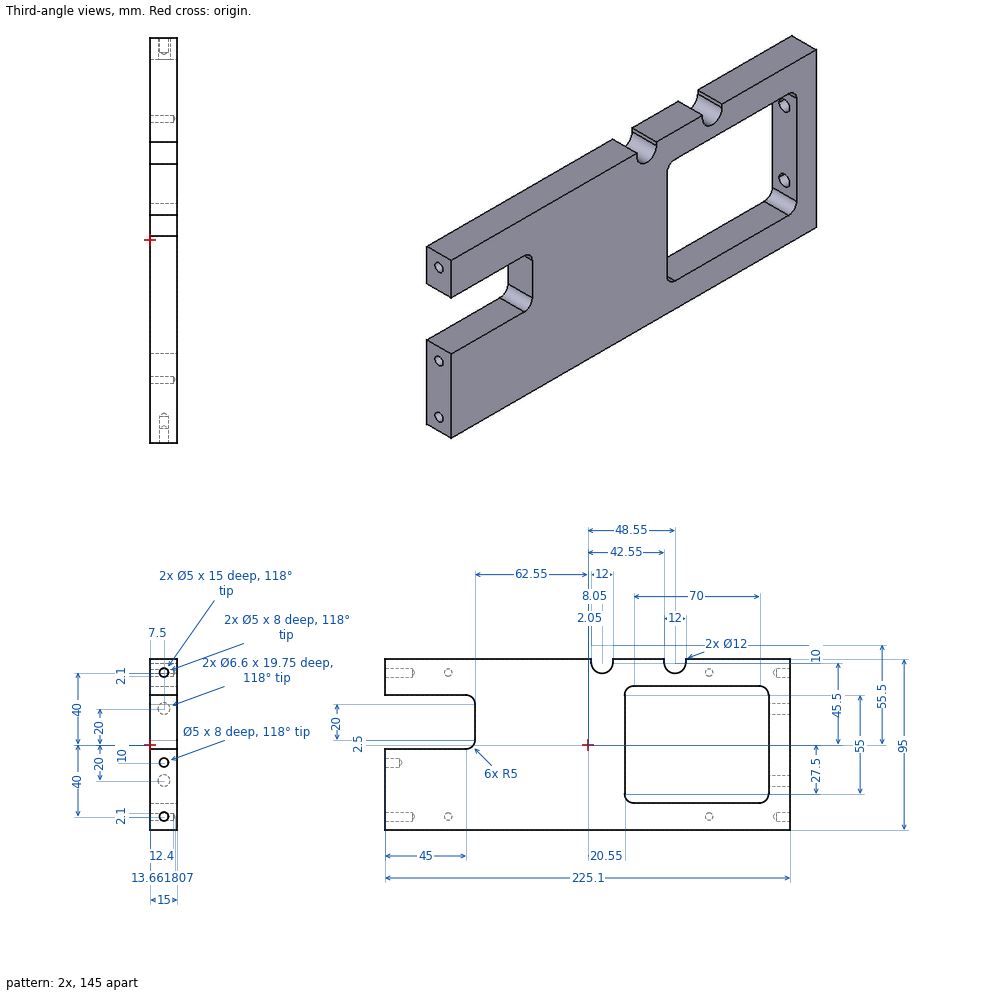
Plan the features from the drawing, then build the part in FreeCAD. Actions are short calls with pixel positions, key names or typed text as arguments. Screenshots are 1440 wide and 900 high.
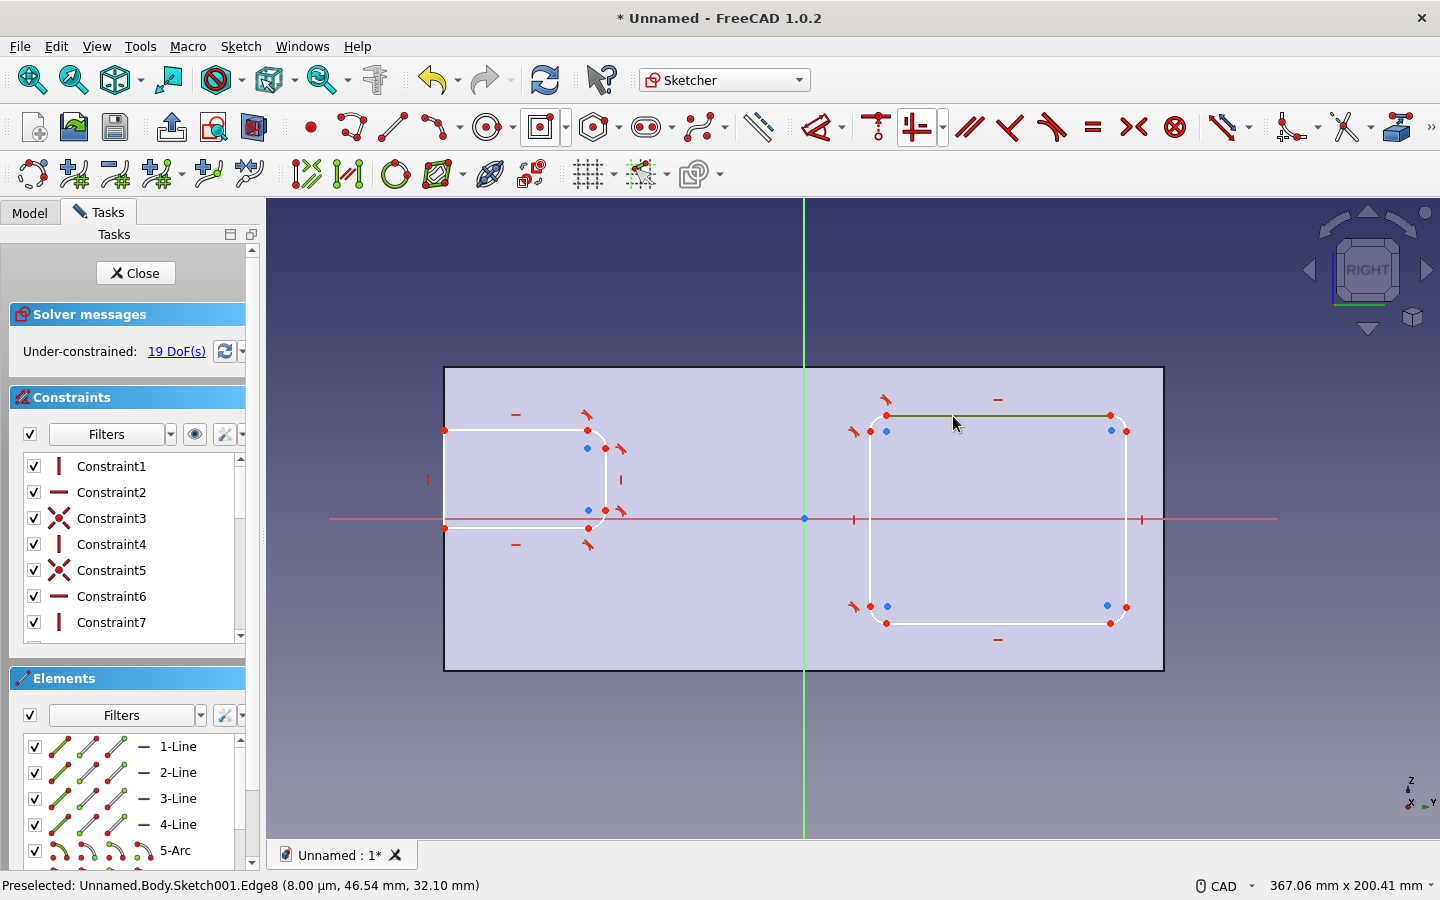
click(1122, 420)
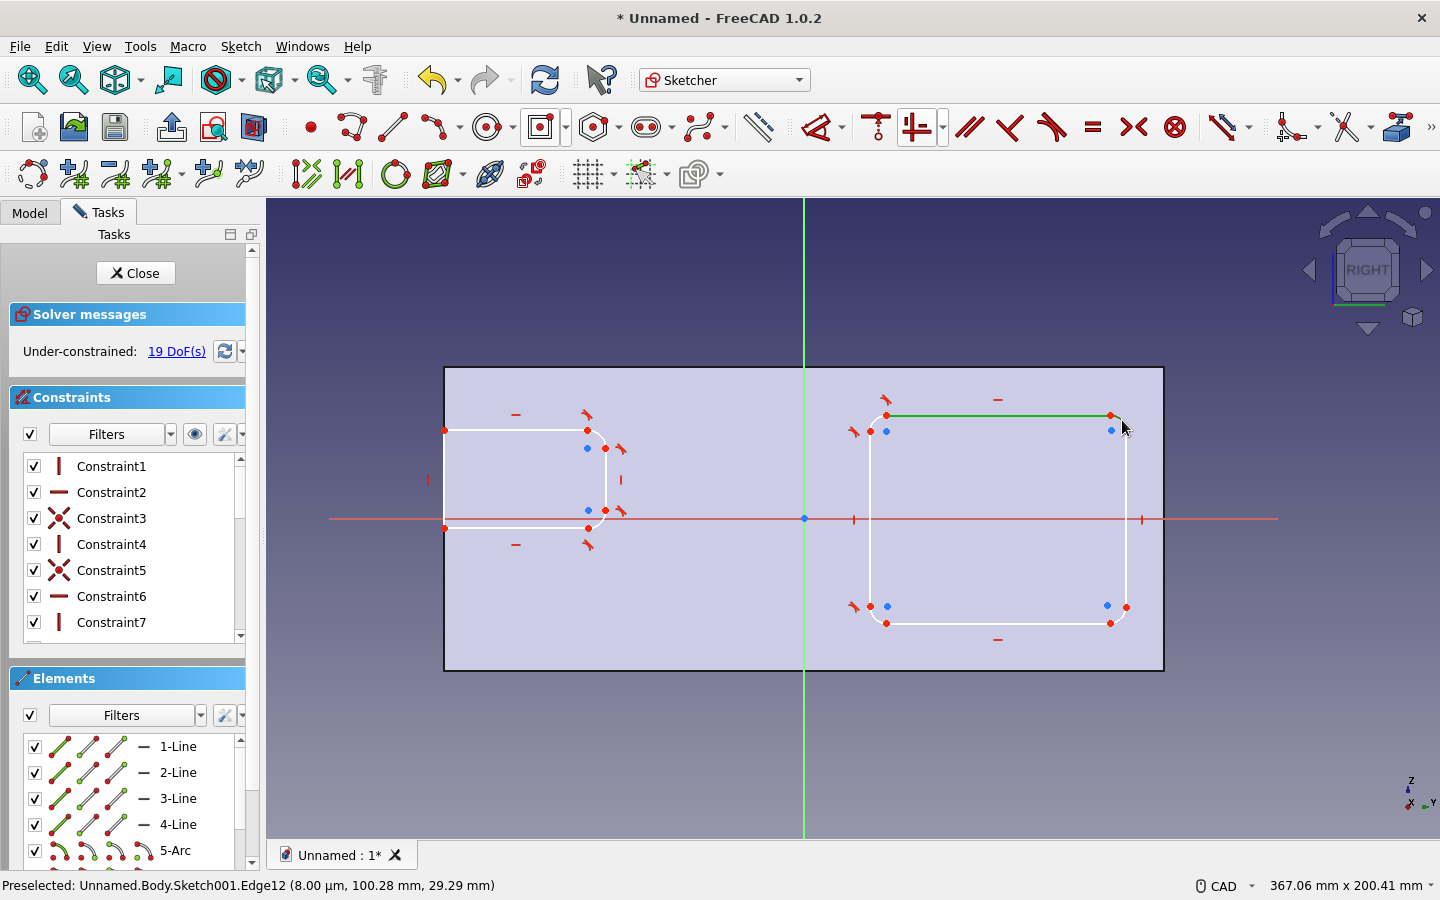
click(1052, 128)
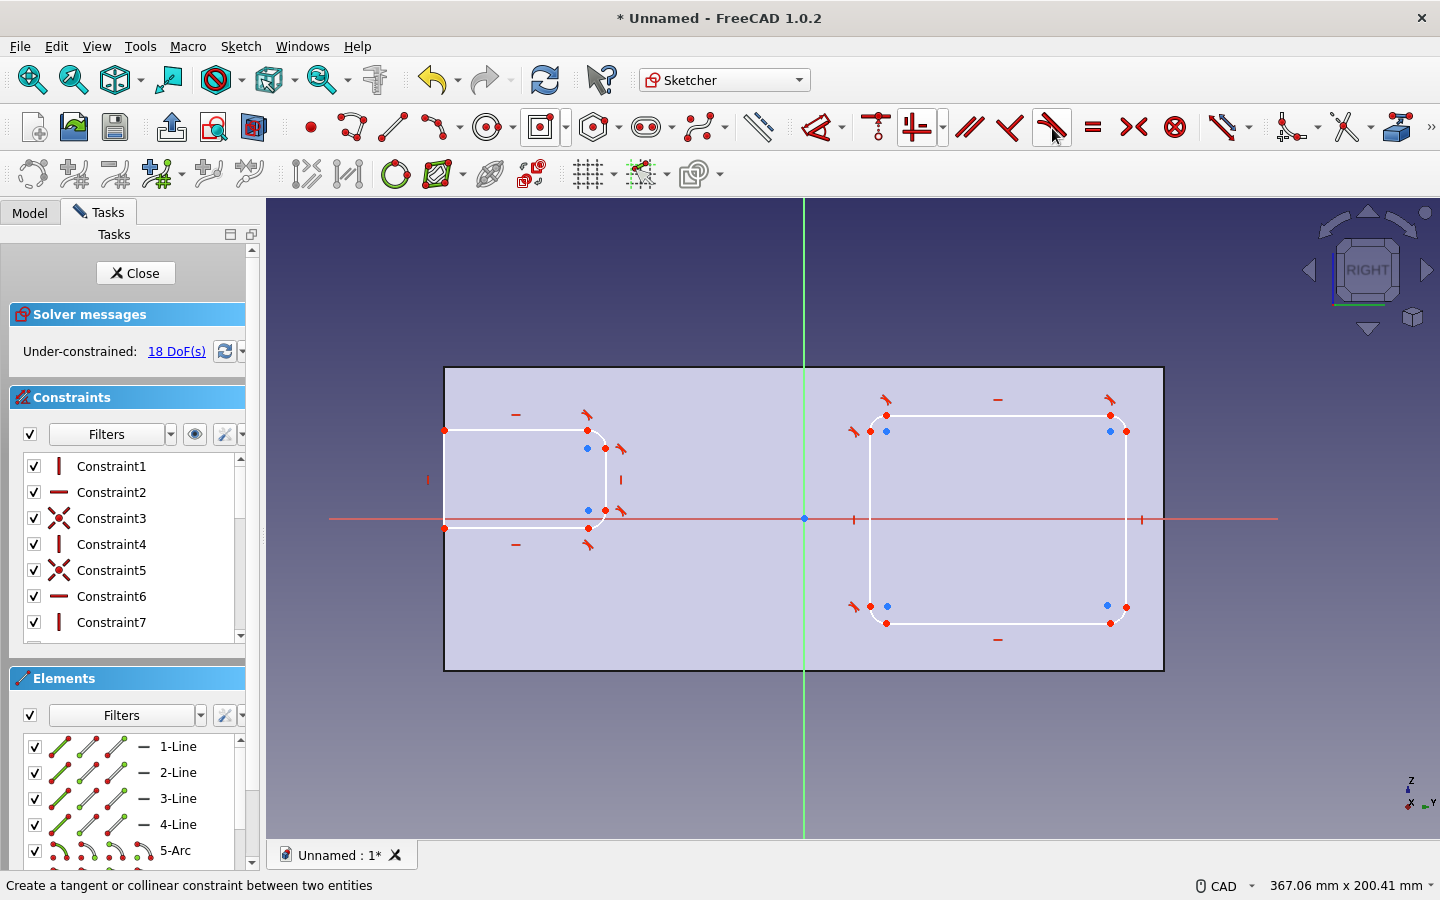
click(1126, 485)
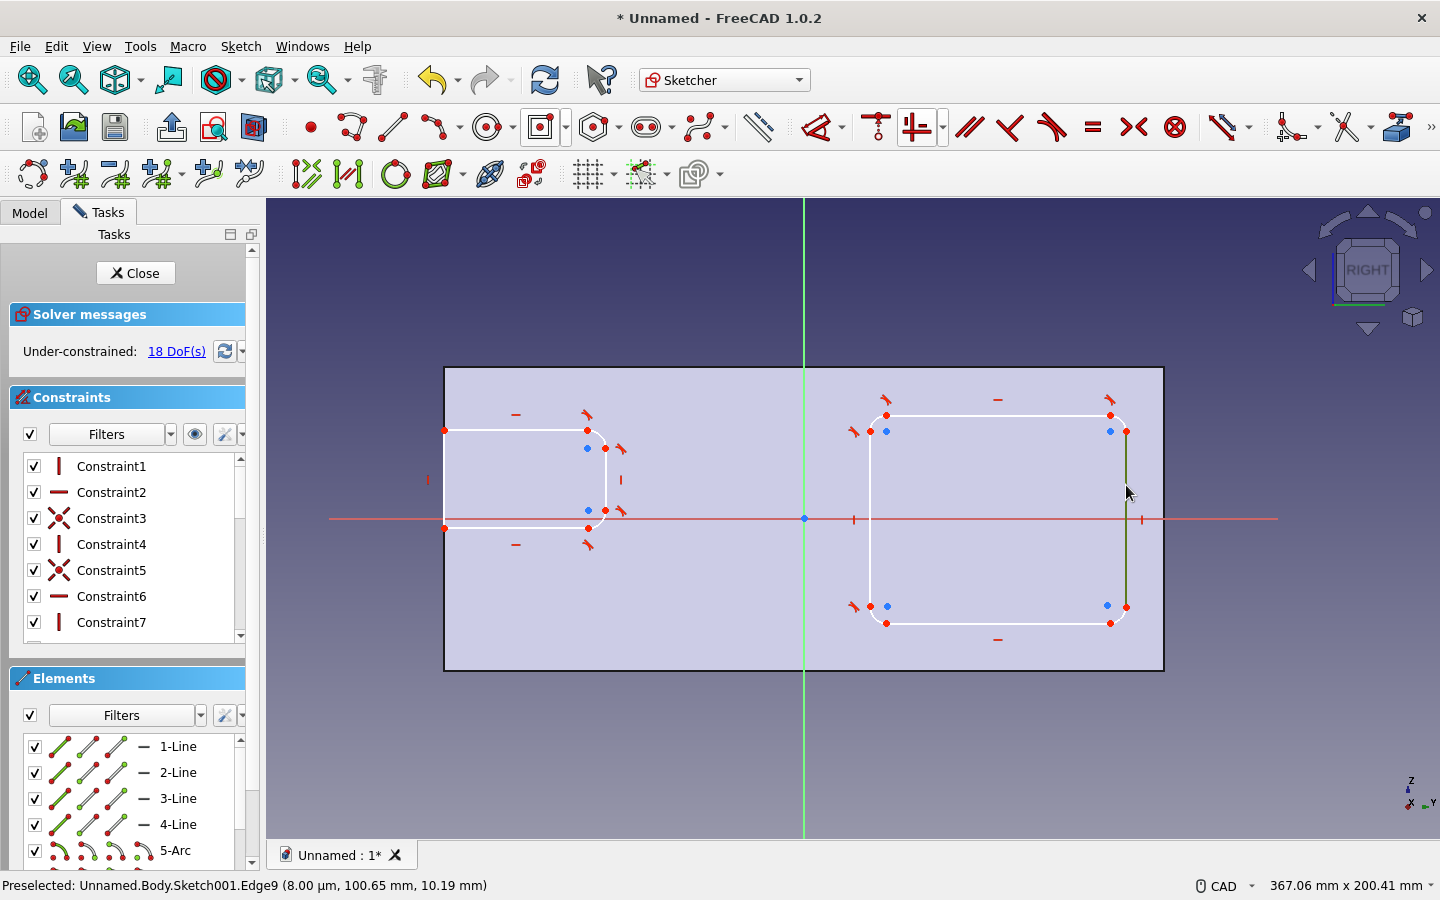
click(1121, 421)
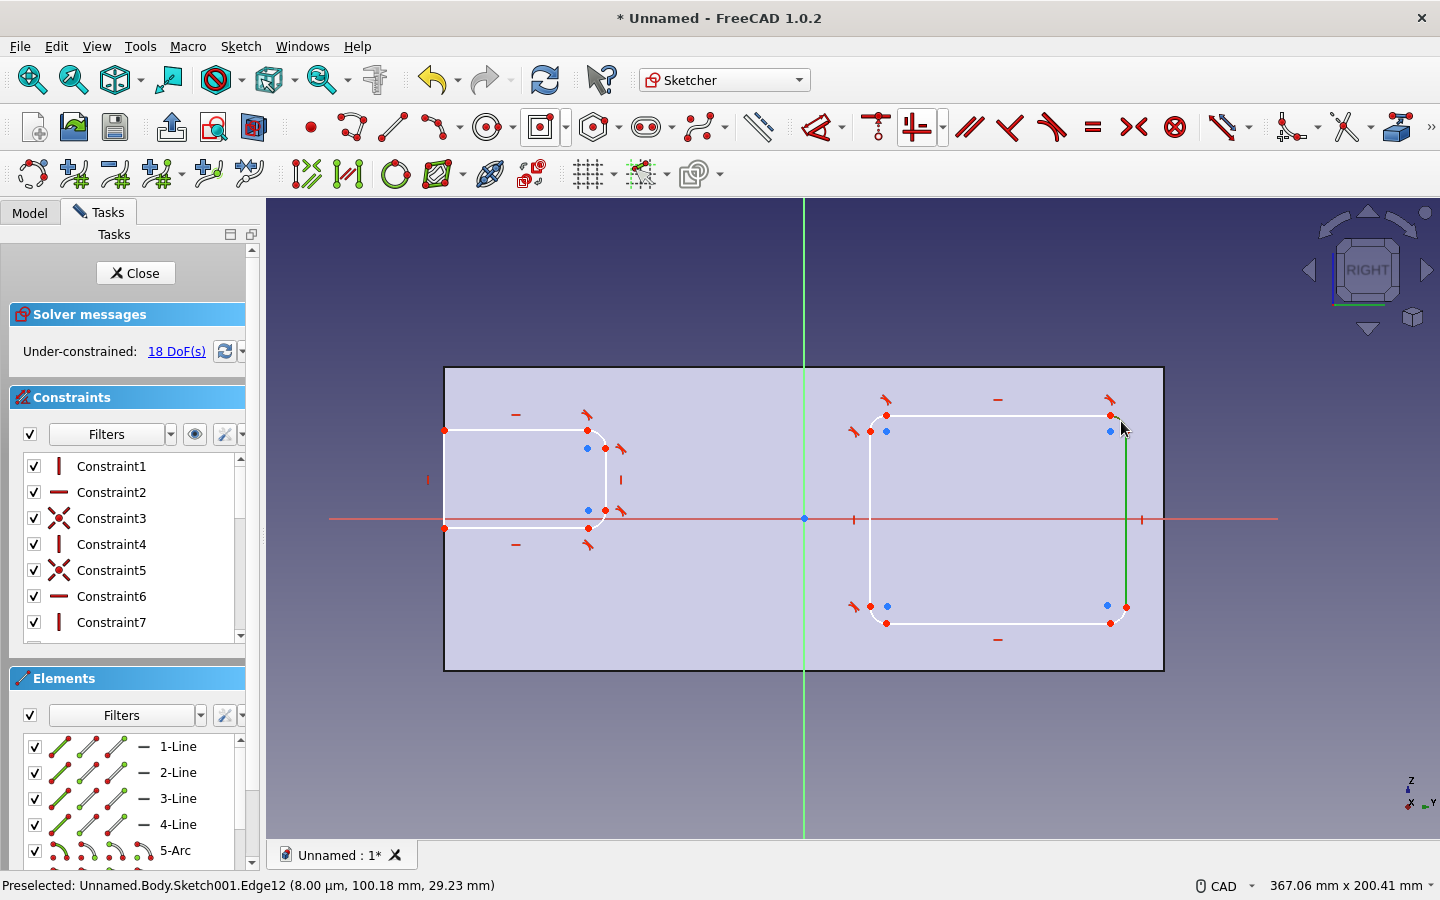
click(1052, 128)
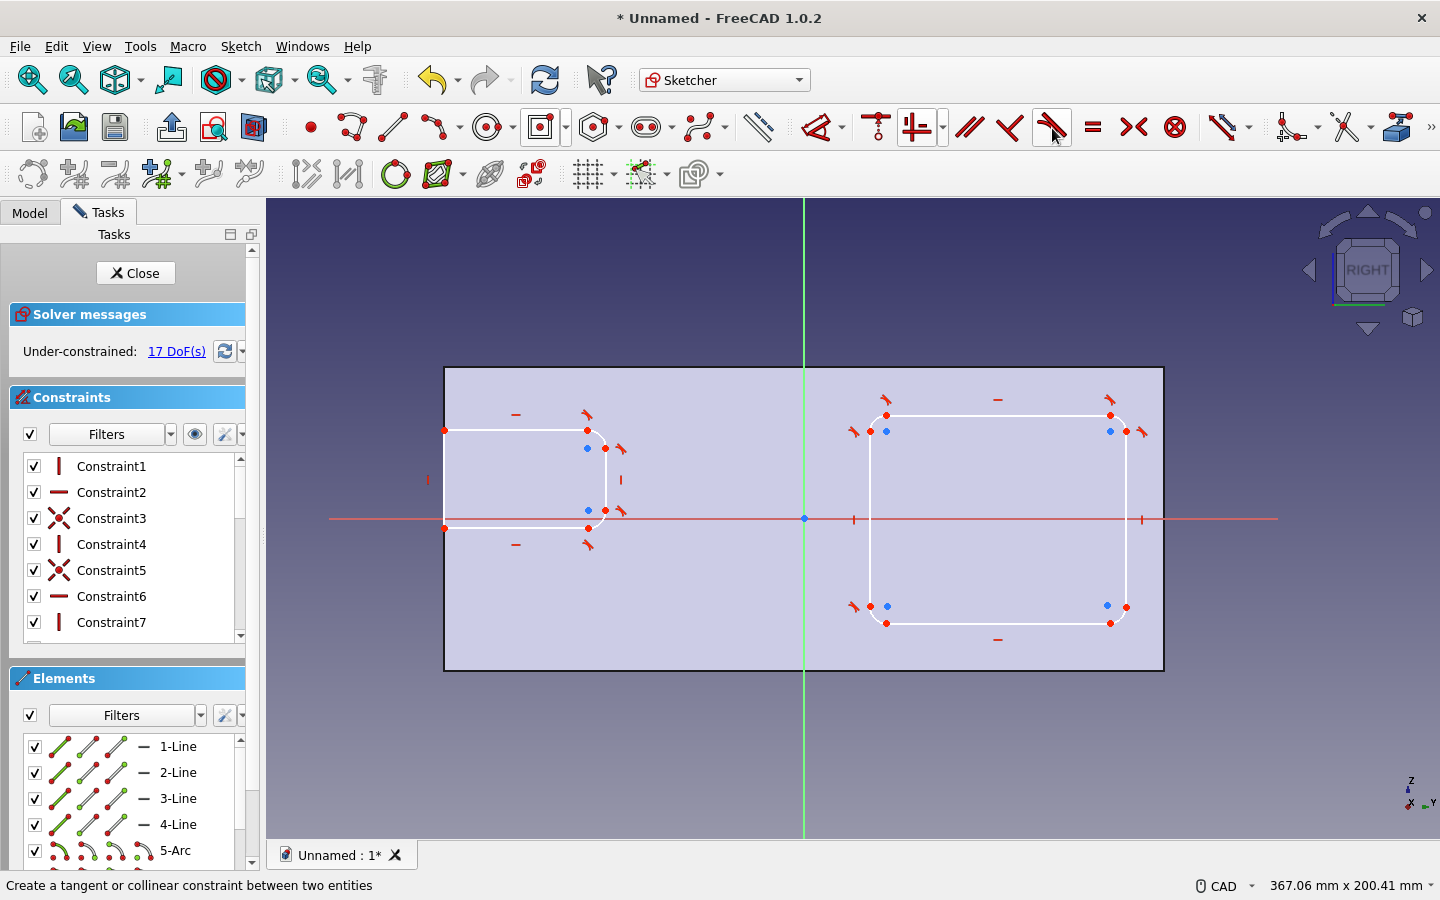
click(1126, 485)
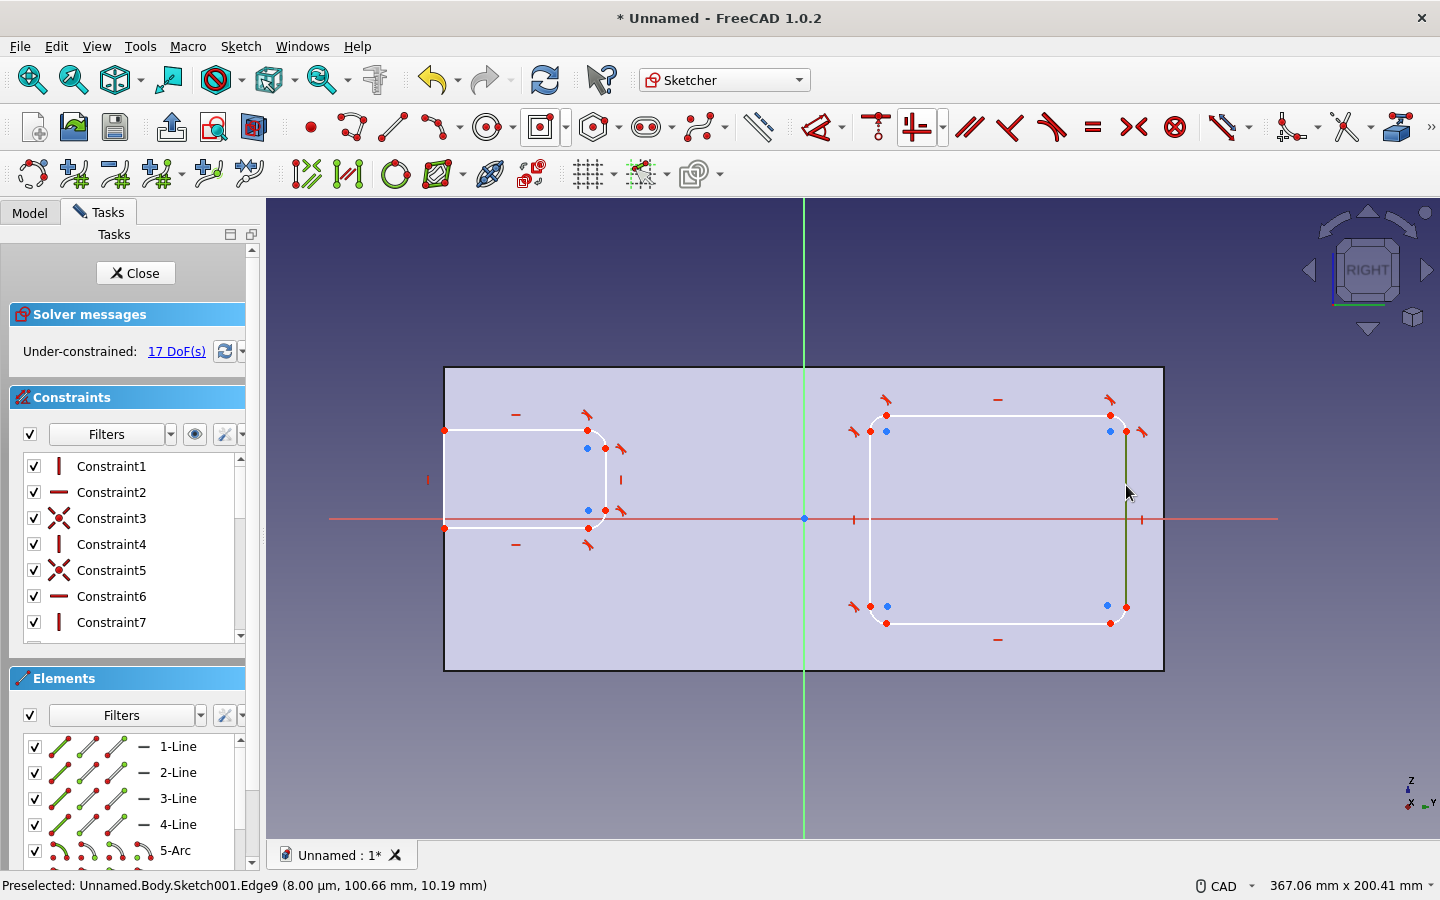
click(1121, 619)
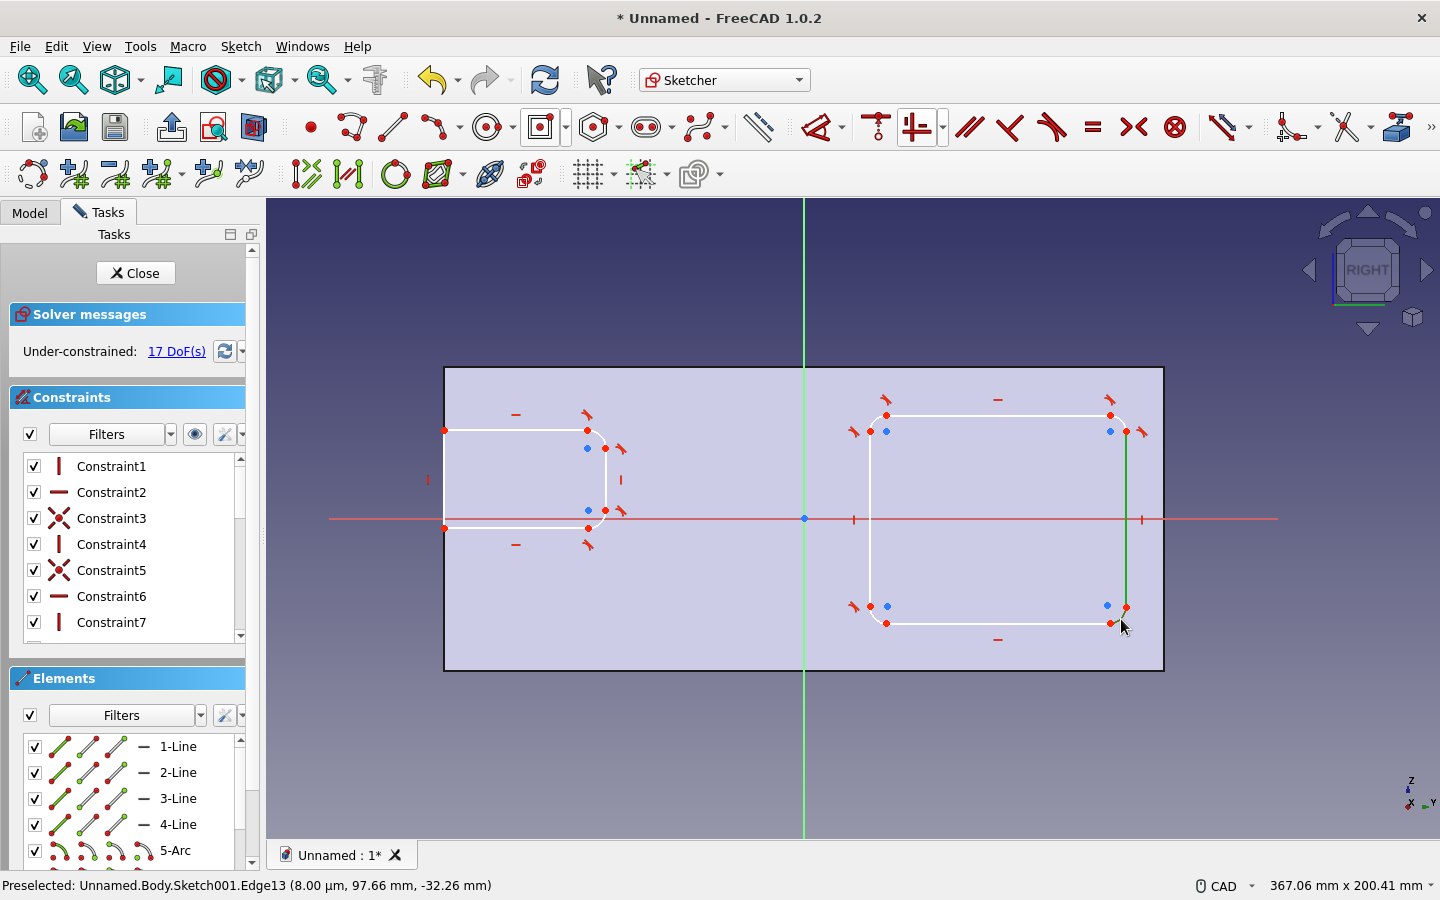
click(1052, 128)